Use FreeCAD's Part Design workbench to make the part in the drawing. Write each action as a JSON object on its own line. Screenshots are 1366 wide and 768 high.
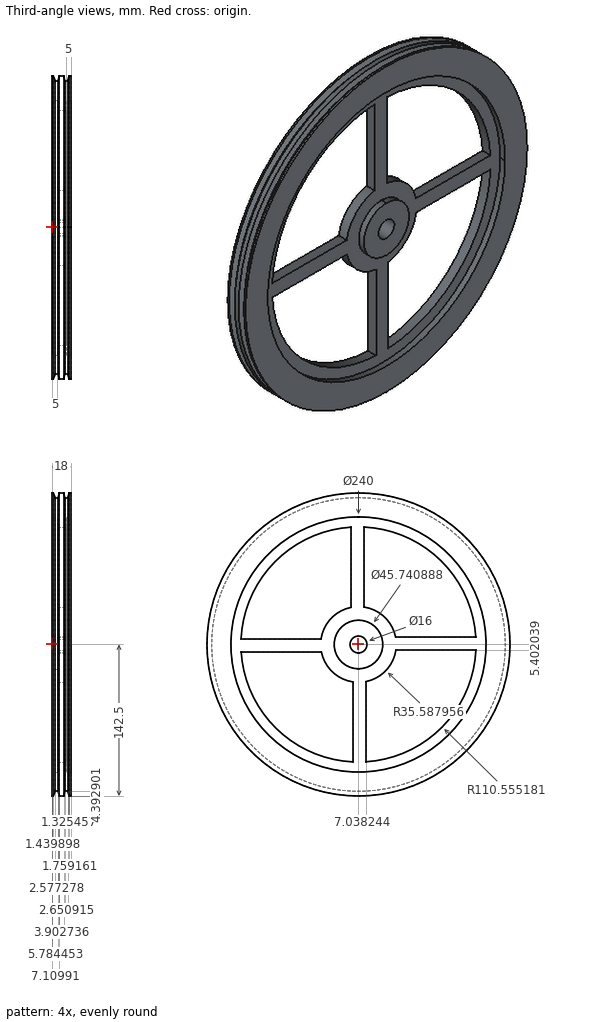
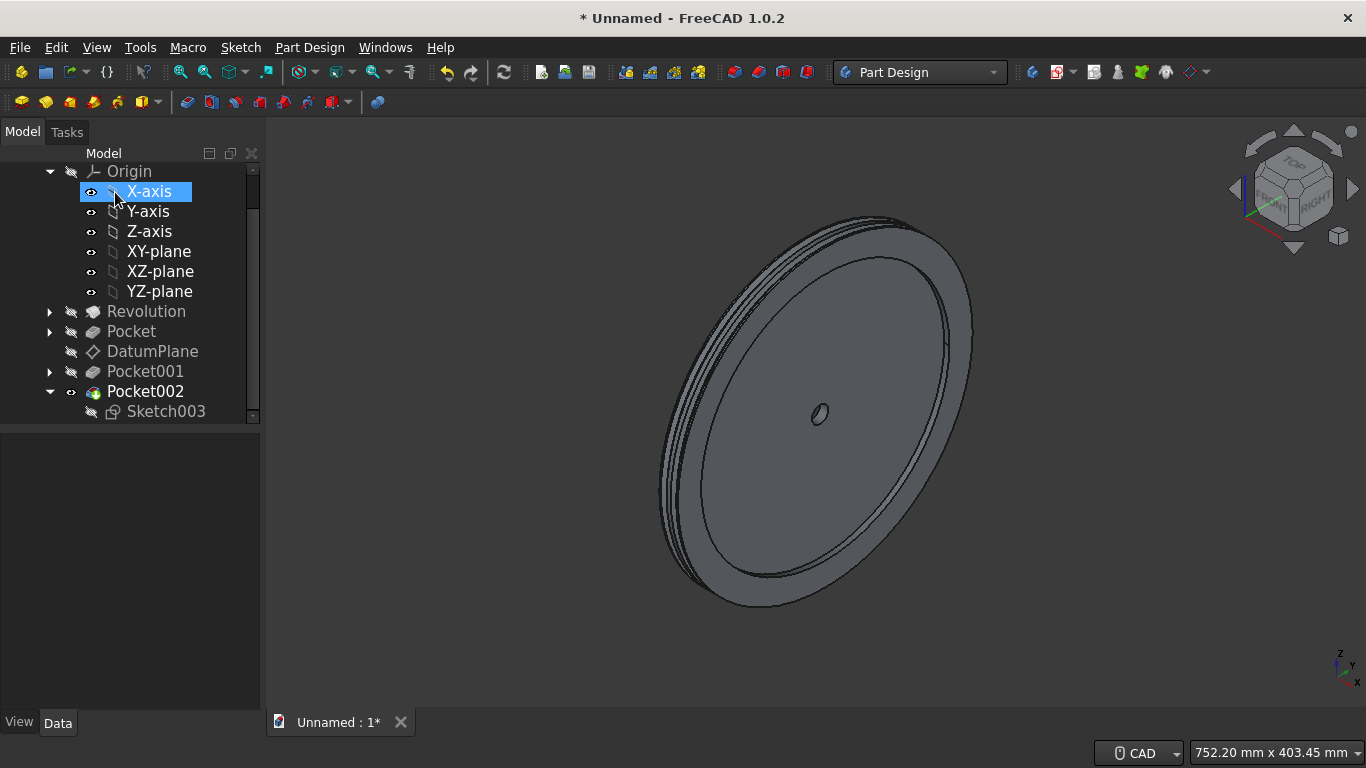
{"action": "left_click", "coordinate": [699, 441]}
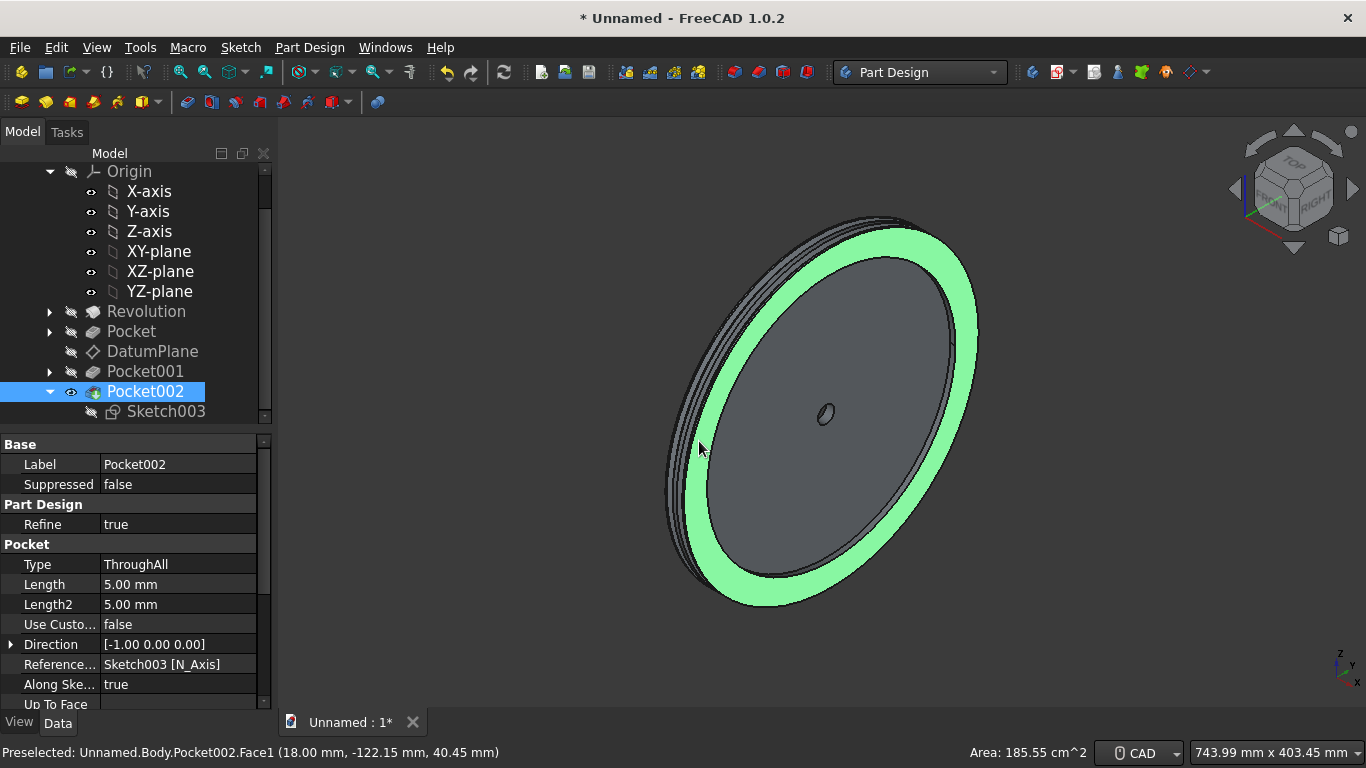
{"action": "left_click", "coordinate": [1058, 72]}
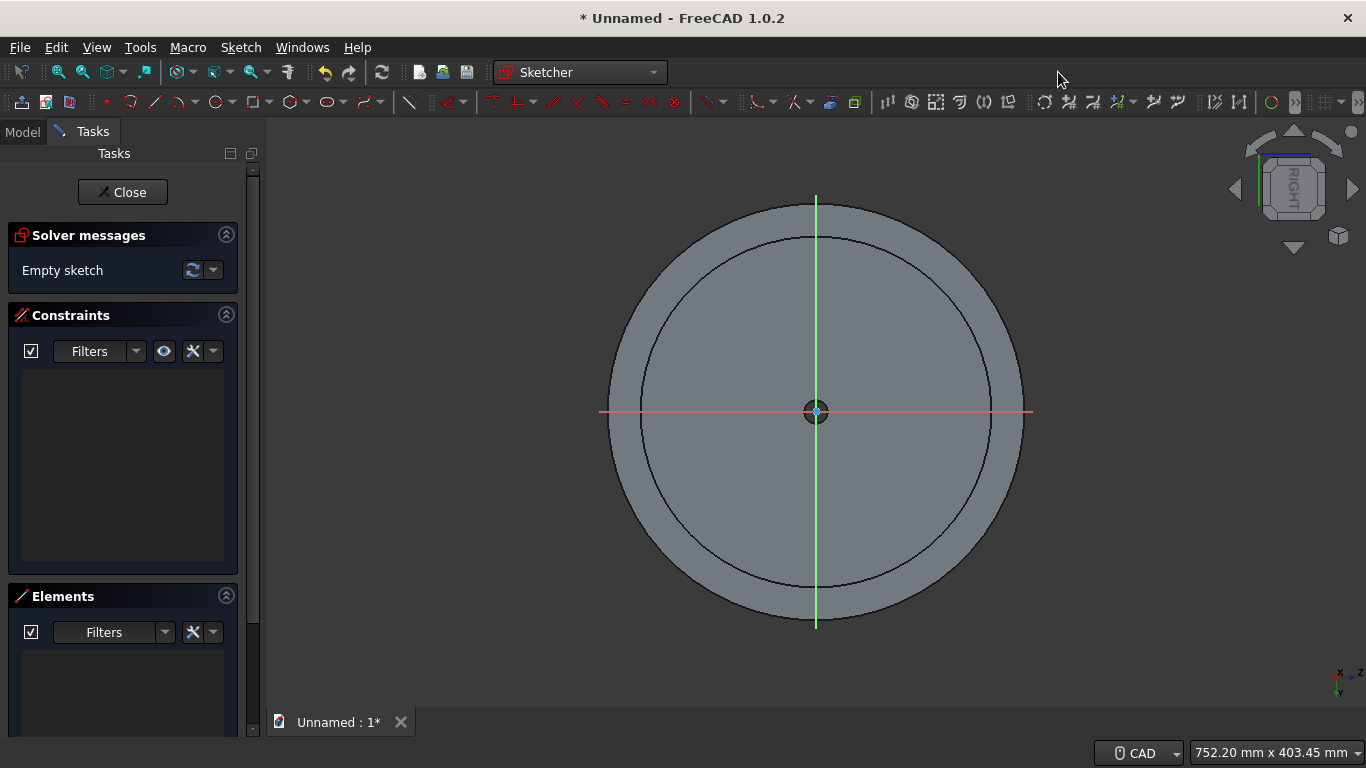
{"action": "scroll", "coordinate": [830, 412], "scroll_direction": "up", "scroll_amount": 9}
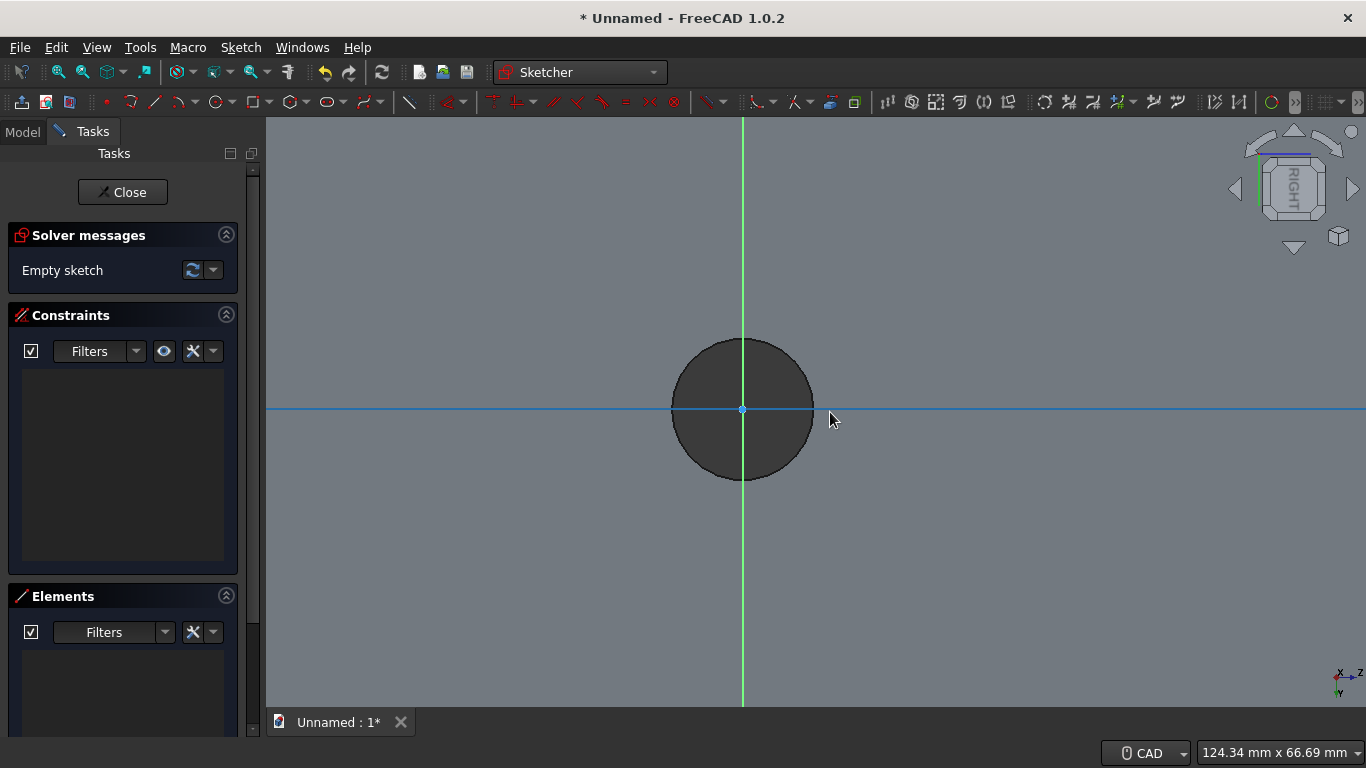
{"action": "key", "text": "g c"}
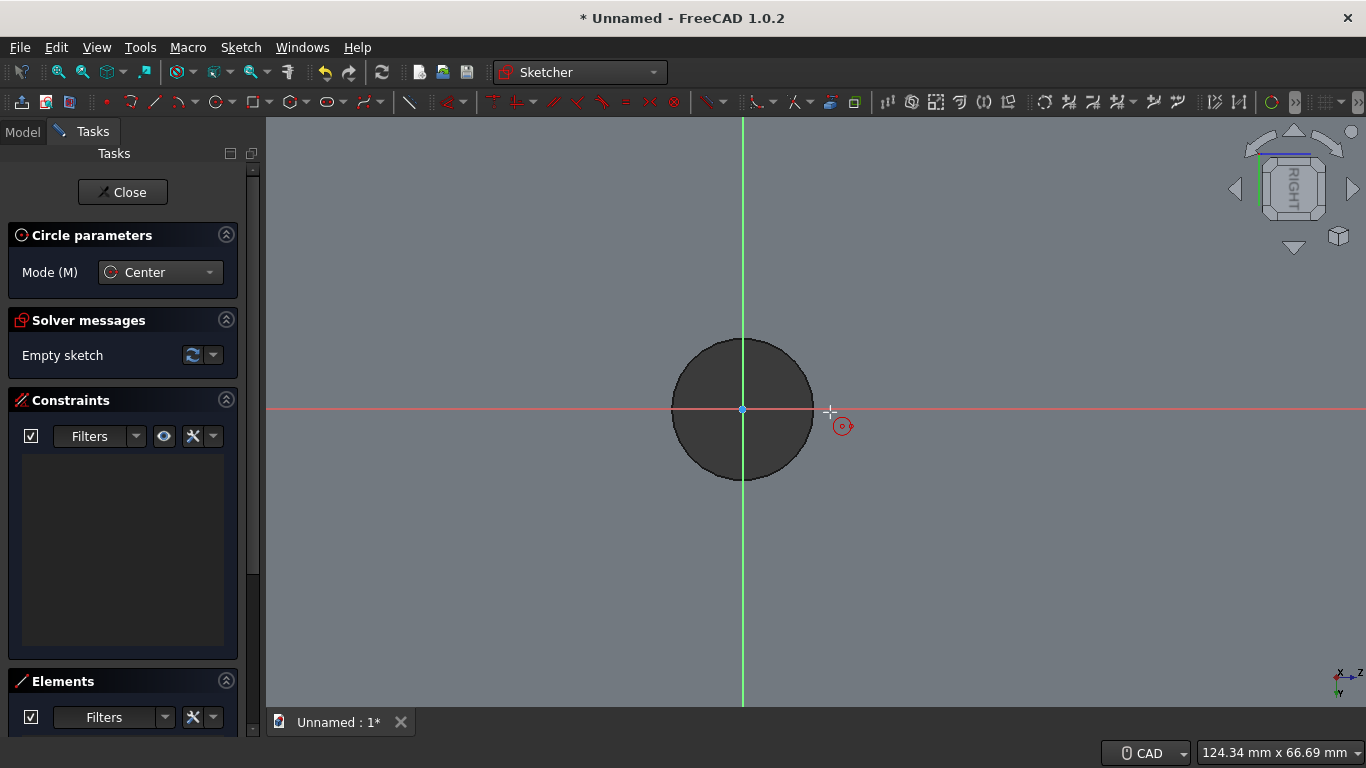
{"action": "left_click", "coordinate": [743, 409]}
{"action": "mouse_move", "coordinate": [886, 266]}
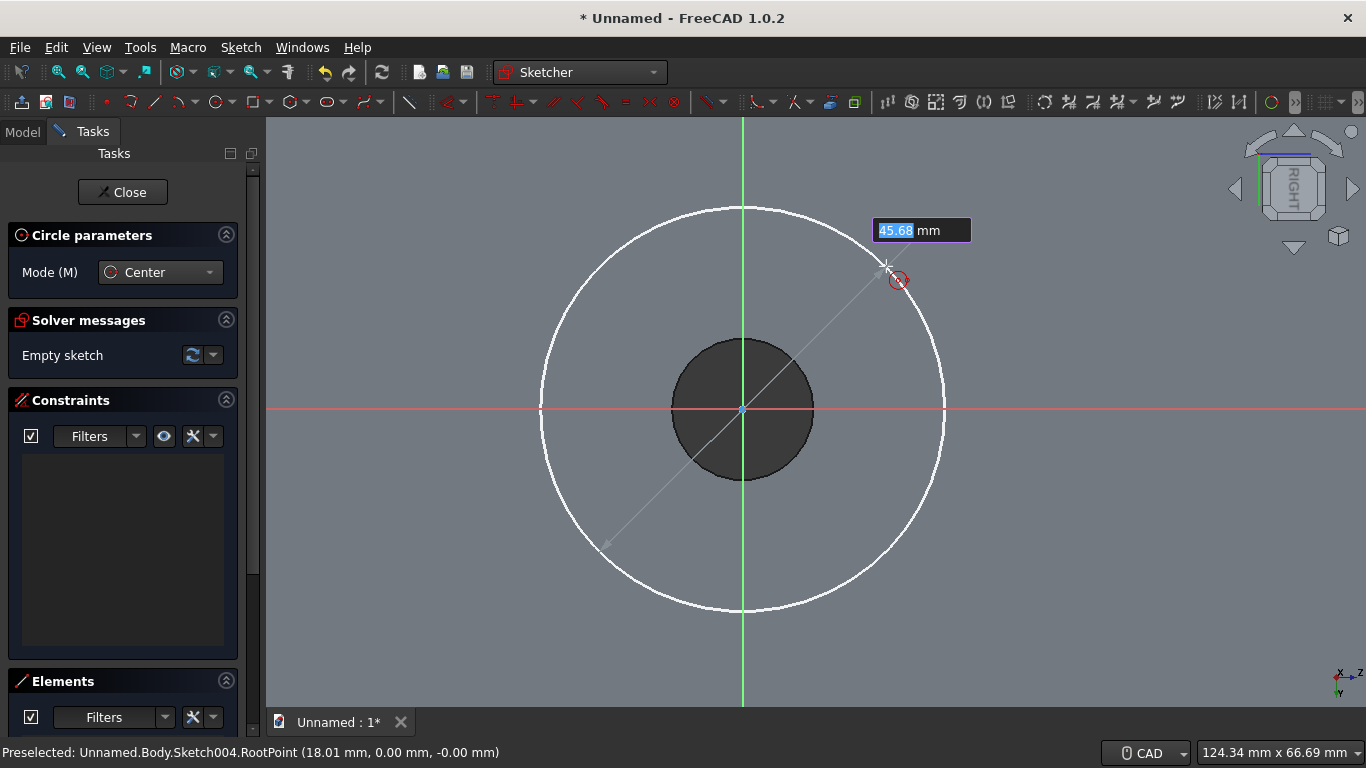
{"action": "type", "text": "45.740888"}
{"action": "key", "text": "Return"}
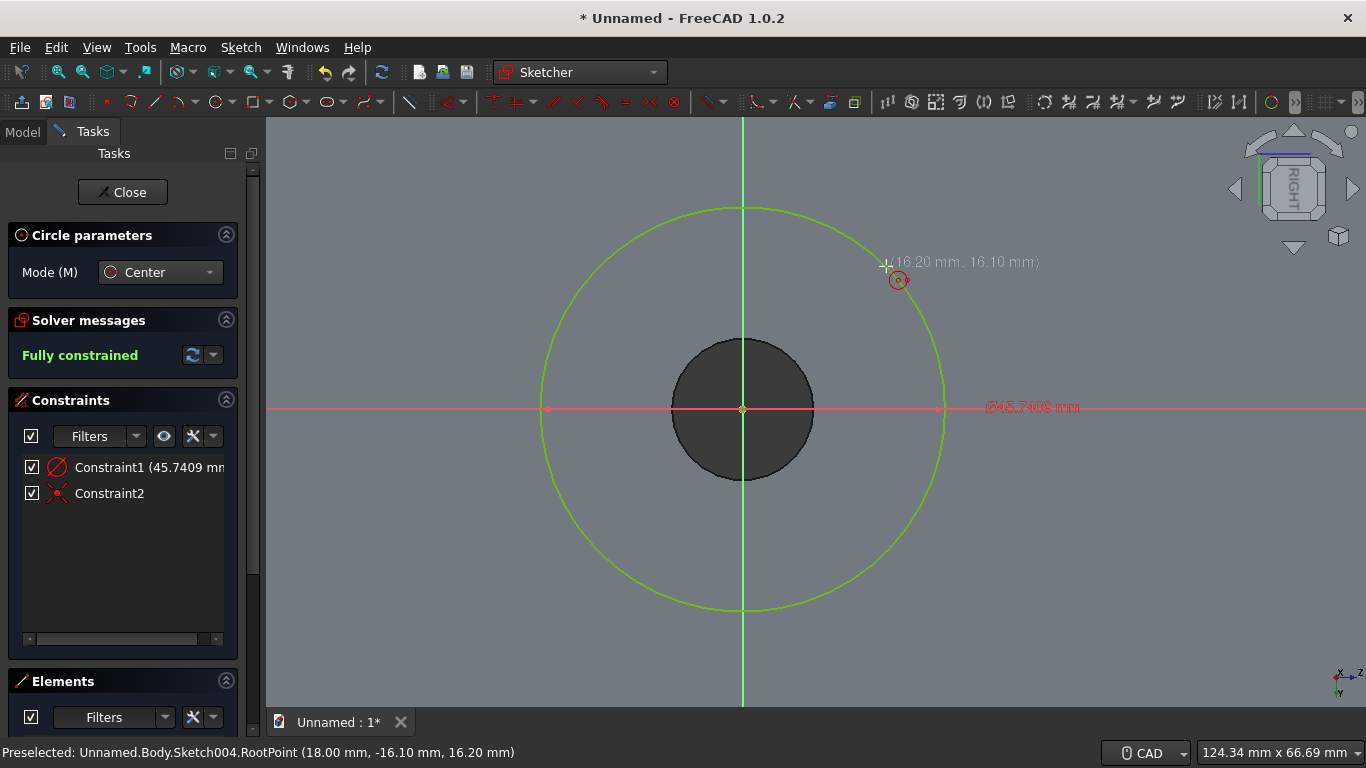
{"action": "left_click", "coordinate": [743, 409]}
{"action": "mouse_move", "coordinate": [793, 359]}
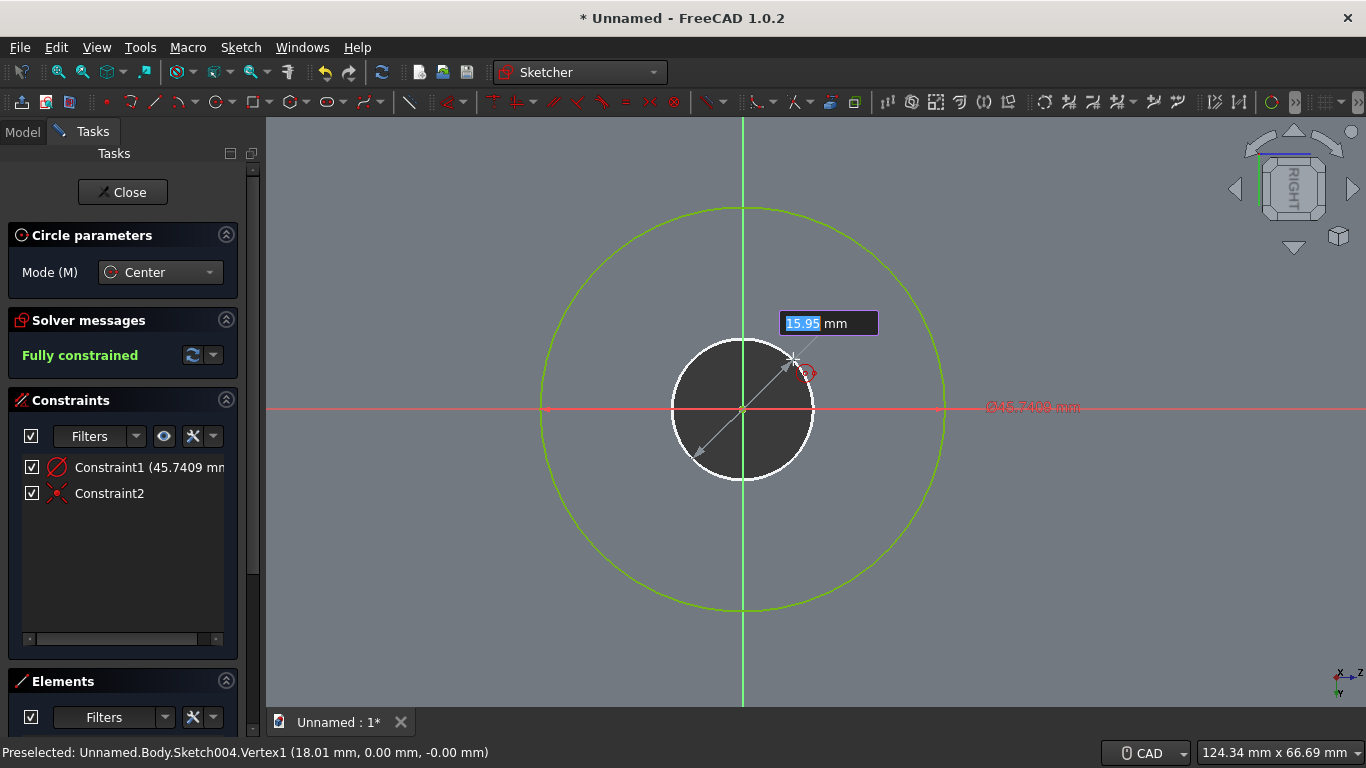
{"action": "type", "text": "16"}
{"action": "key", "text": "Return"}
{"action": "key", "text": "Escape"}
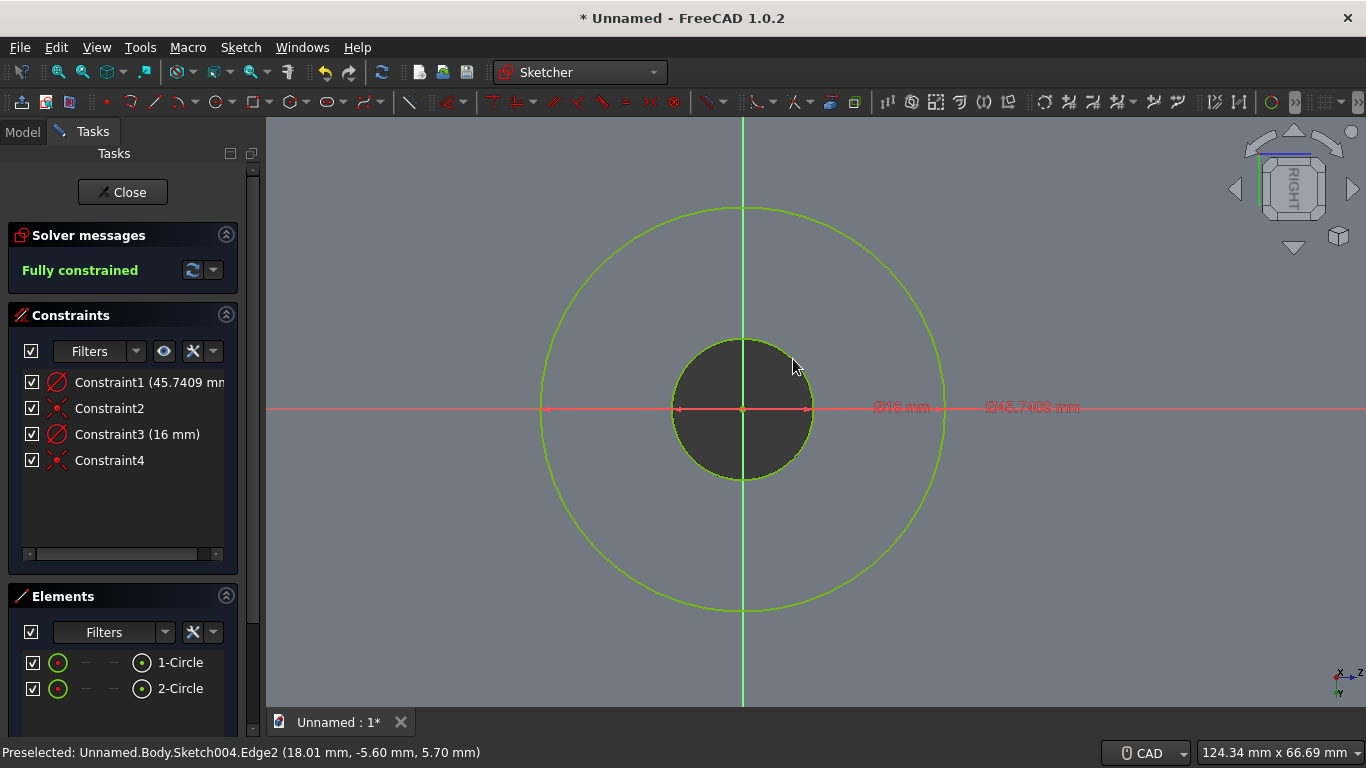
{"action": "left_click", "coordinate": [123, 192]}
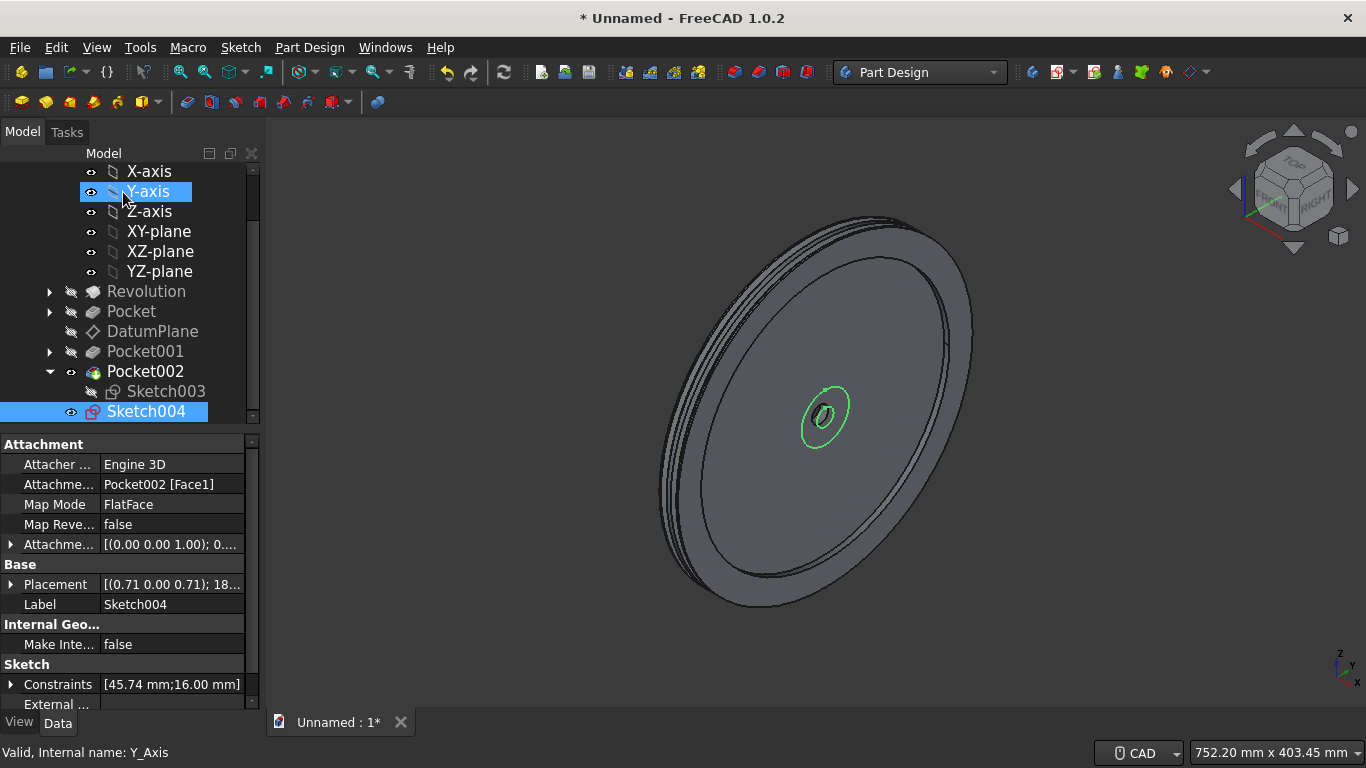
{"action": "left_click", "coordinate": [22, 102]}